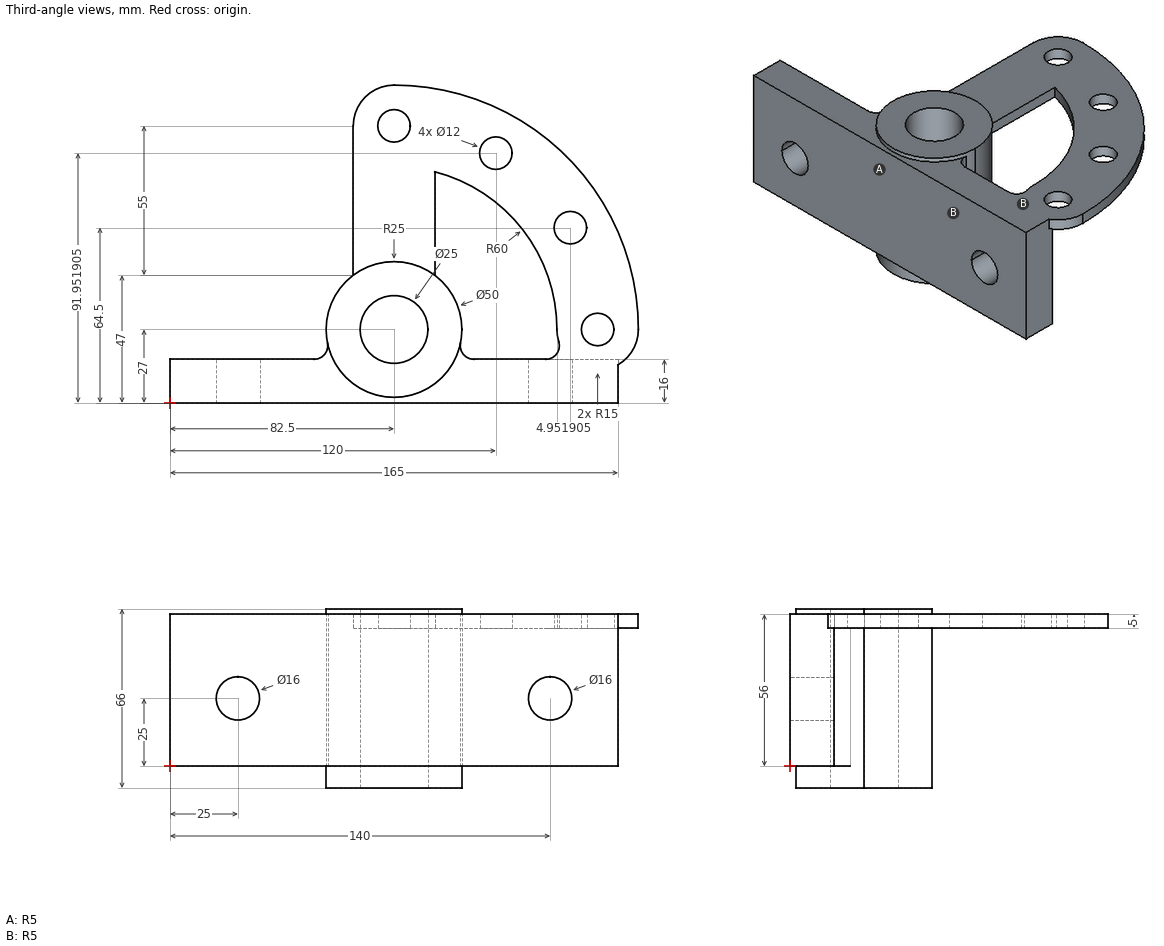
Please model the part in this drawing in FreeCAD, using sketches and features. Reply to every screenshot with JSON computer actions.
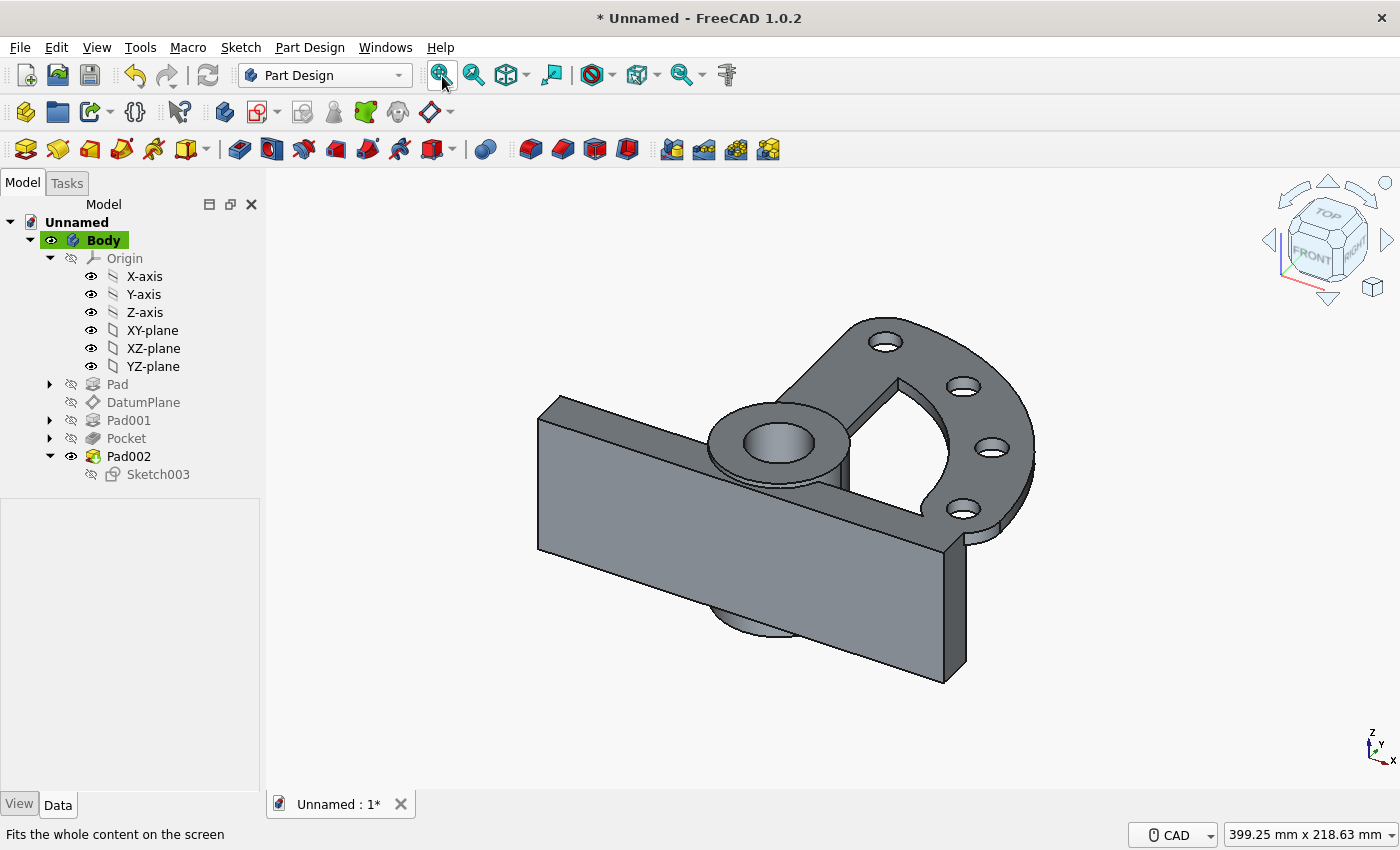
{"action": "key", "text": "4"}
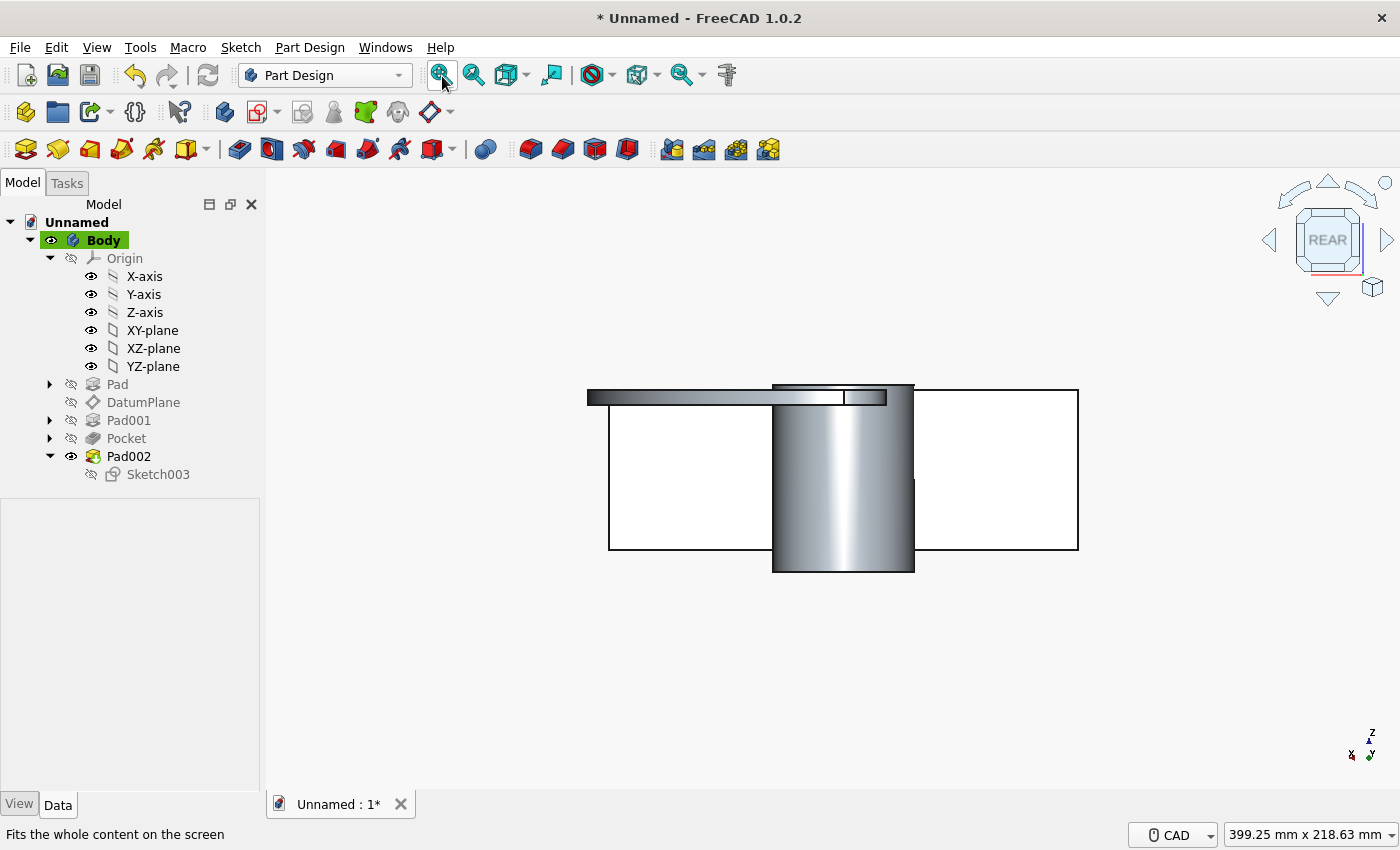
{"action": "left_click", "coordinate": [442, 76]}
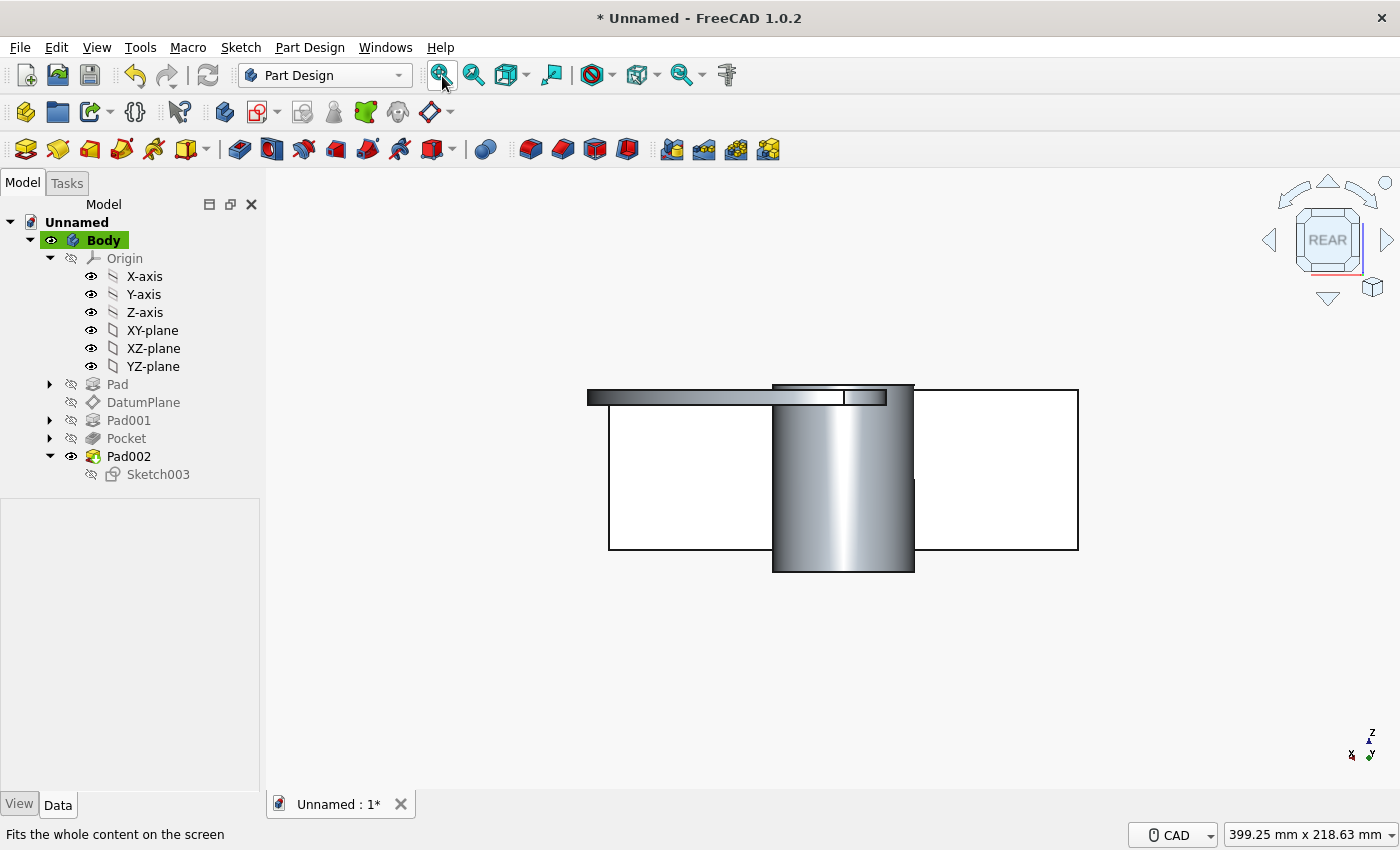
{"action": "left_click", "coordinate": [993, 469]}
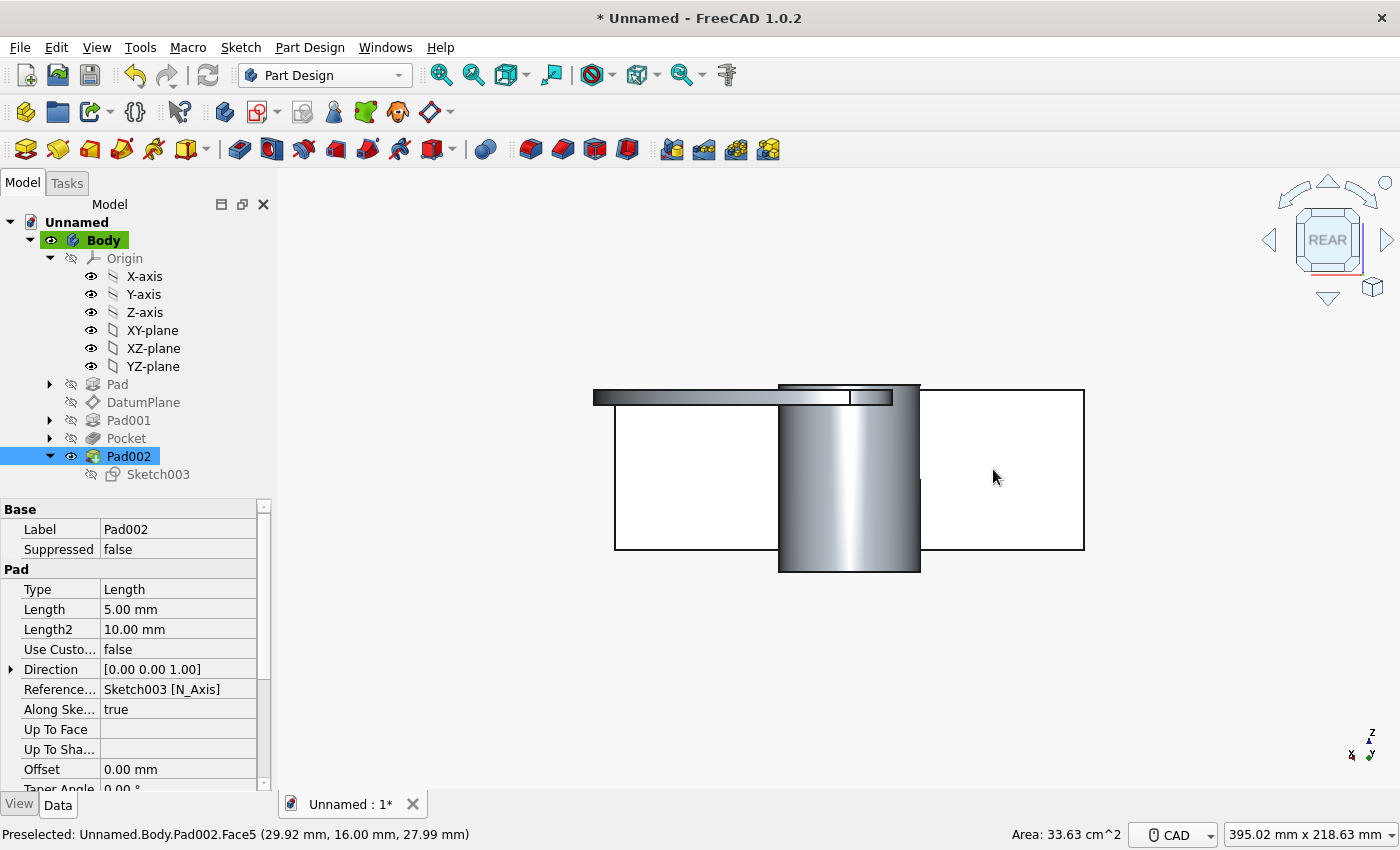
{"action": "left_click", "coordinate": [258, 112]}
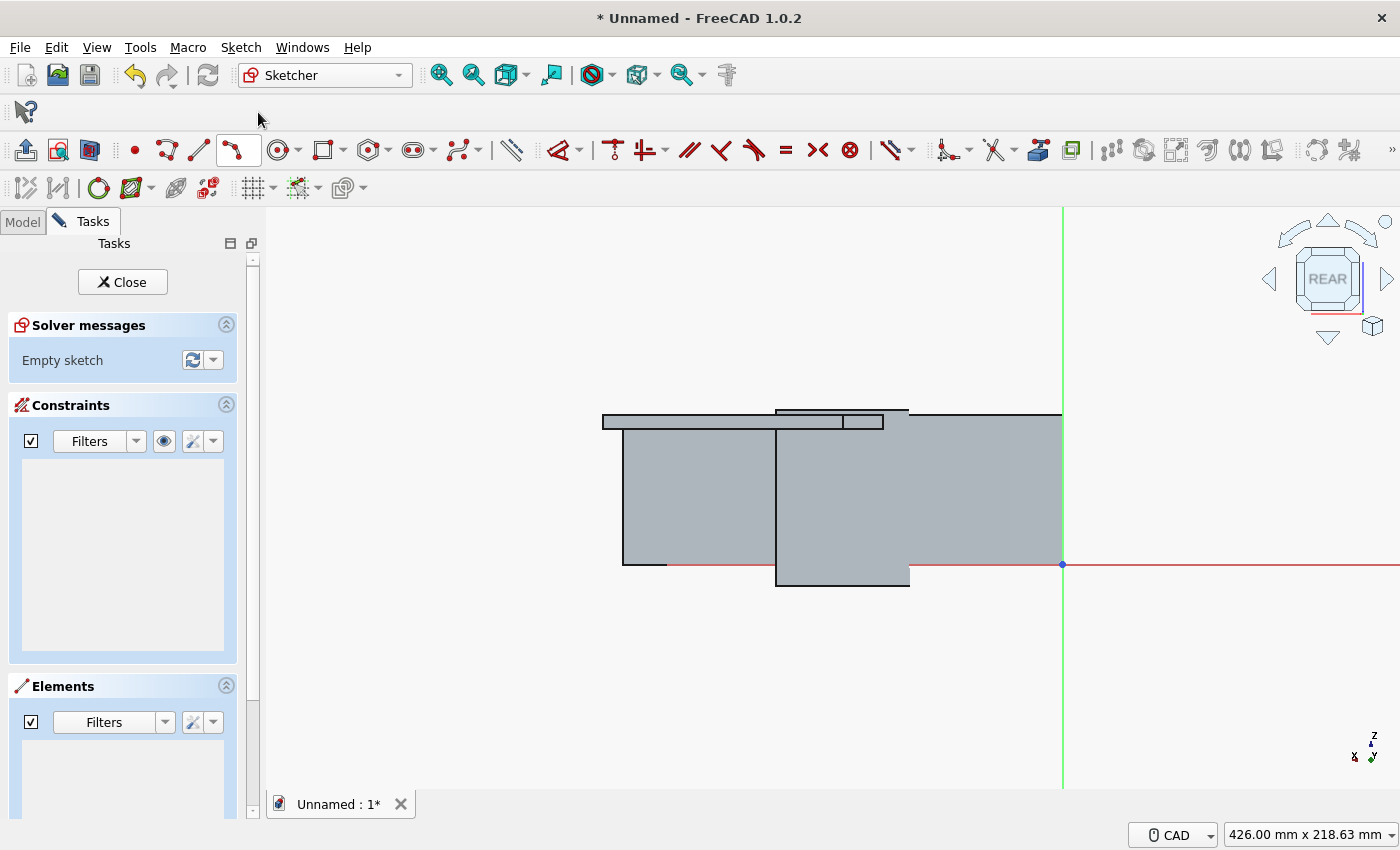
{"action": "left_click", "coordinate": [90, 150]}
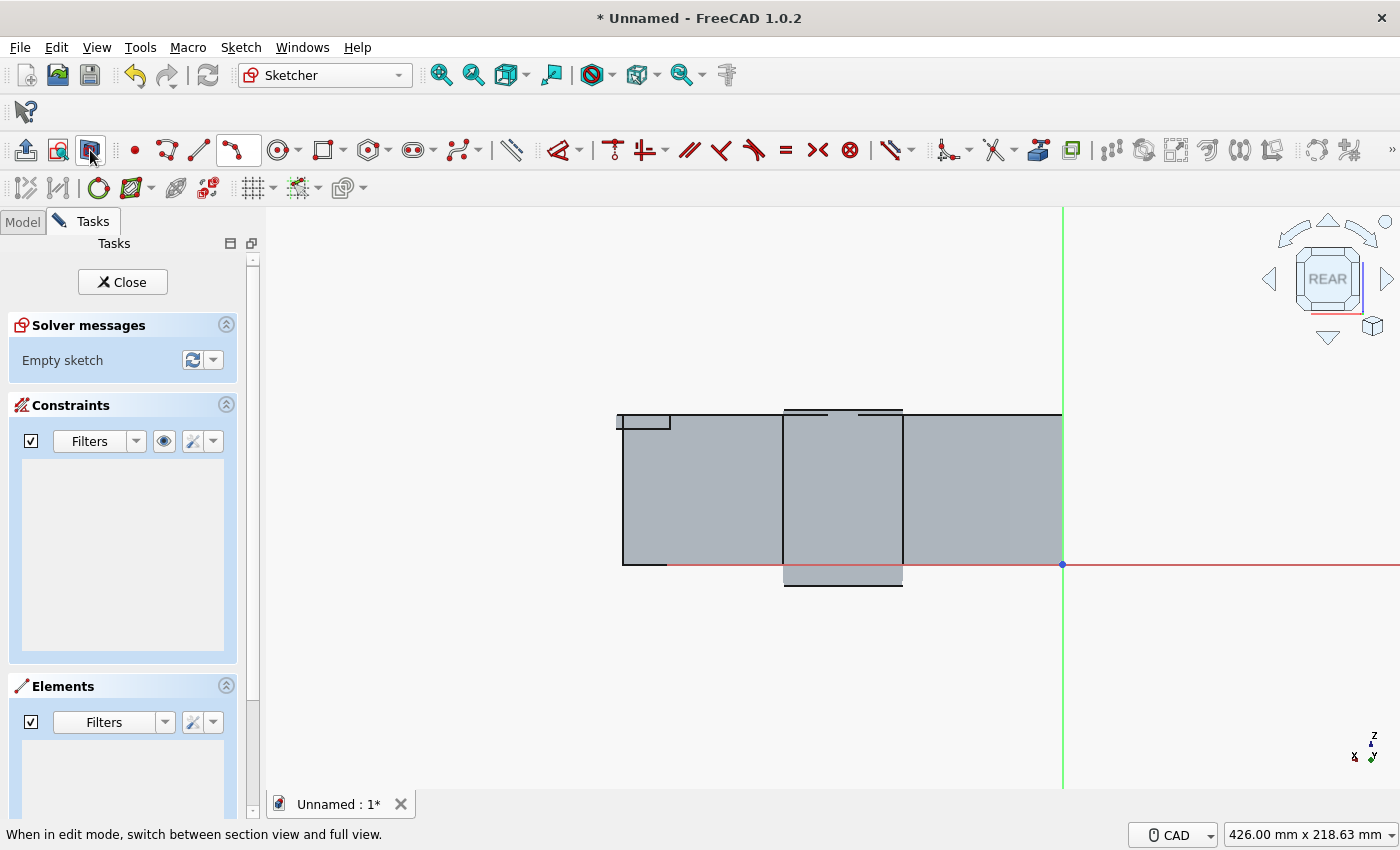
{"action": "scroll", "coordinate": [1102, 528], "scroll_direction": "up", "scroll_amount": 7}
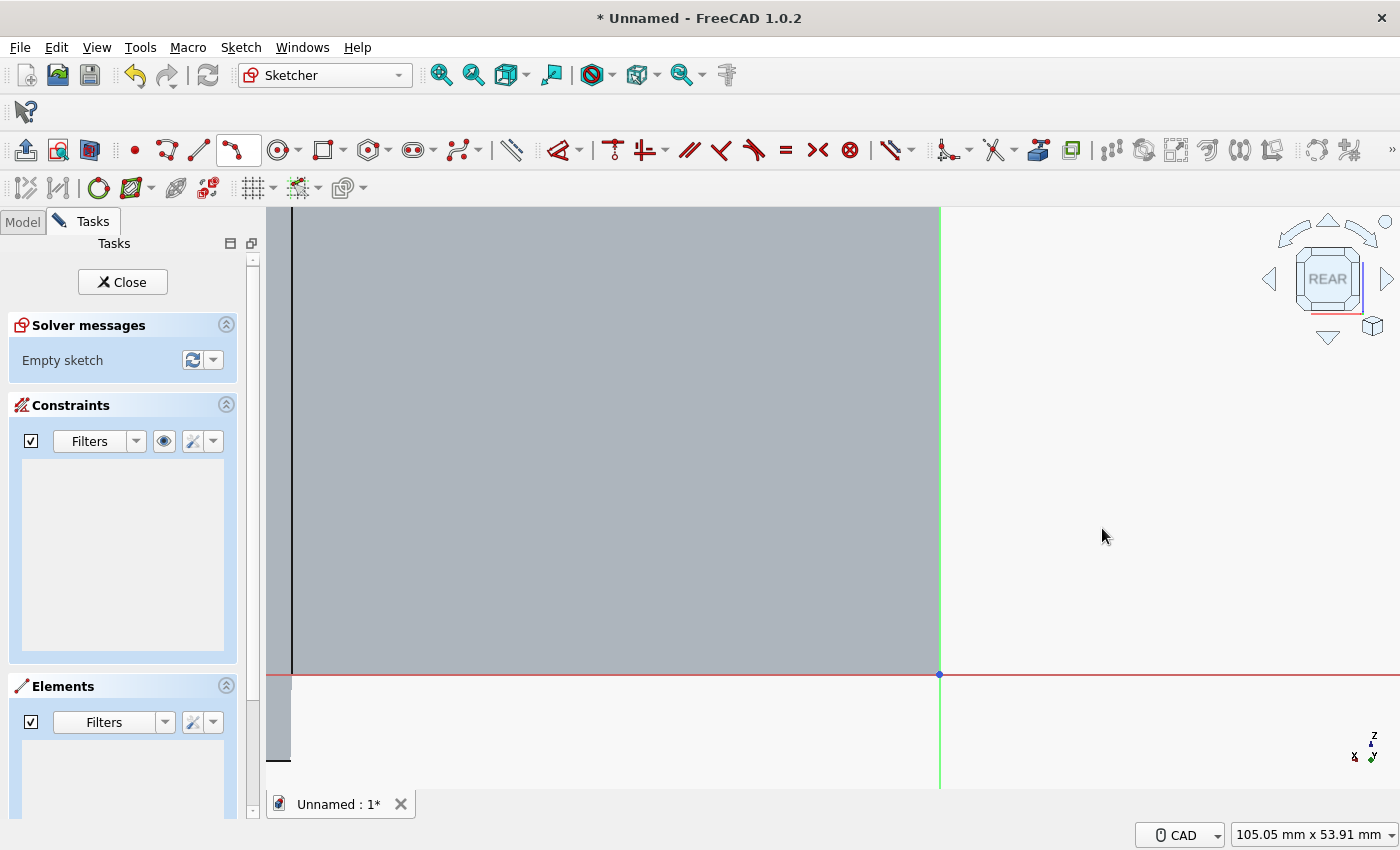
{"action": "key", "text": "g c"}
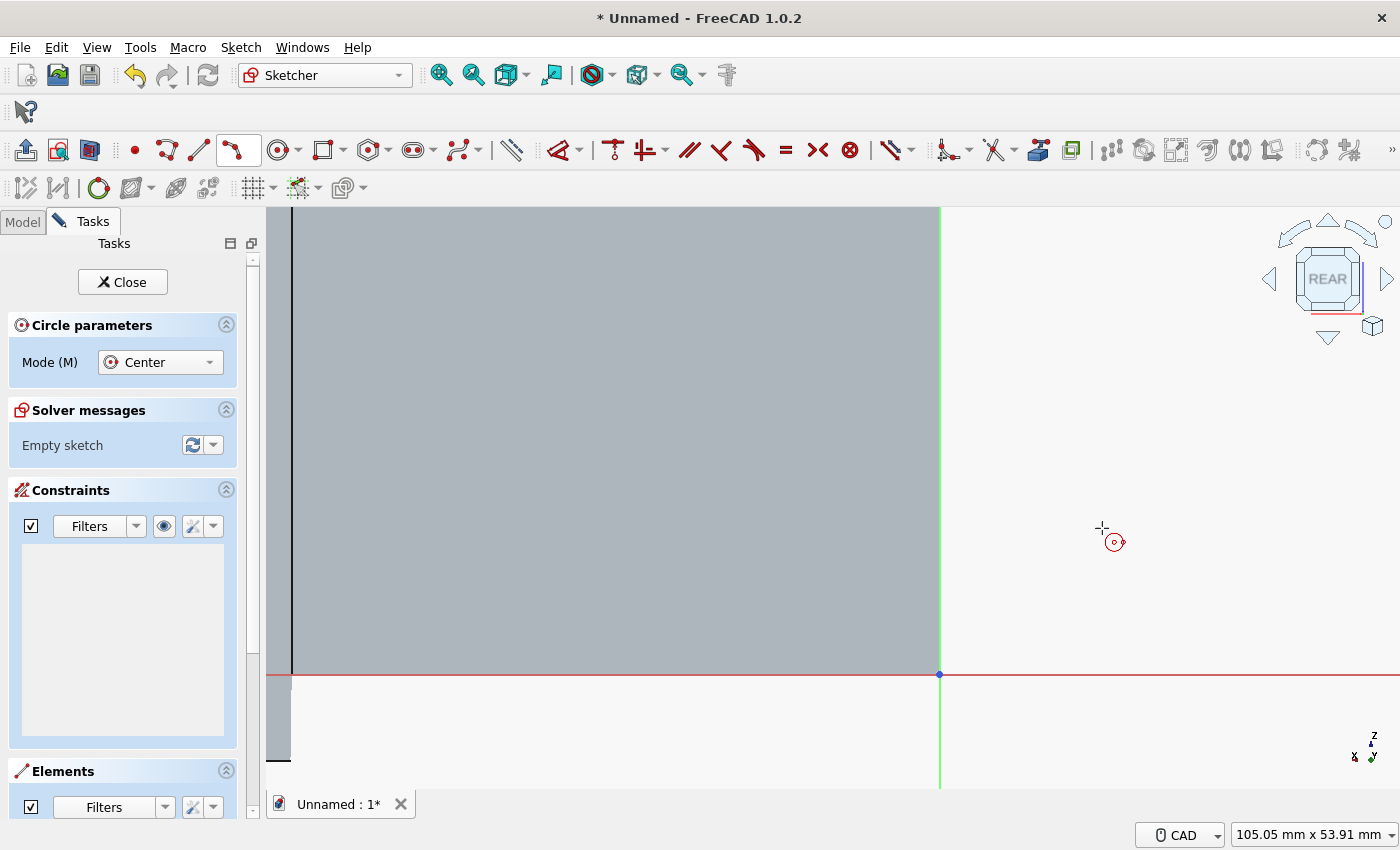
{"action": "left_click", "coordinate": [670, 405]}
{"action": "left_click", "coordinate": [731, 344]}
{"action": "key", "text": "Escape"}